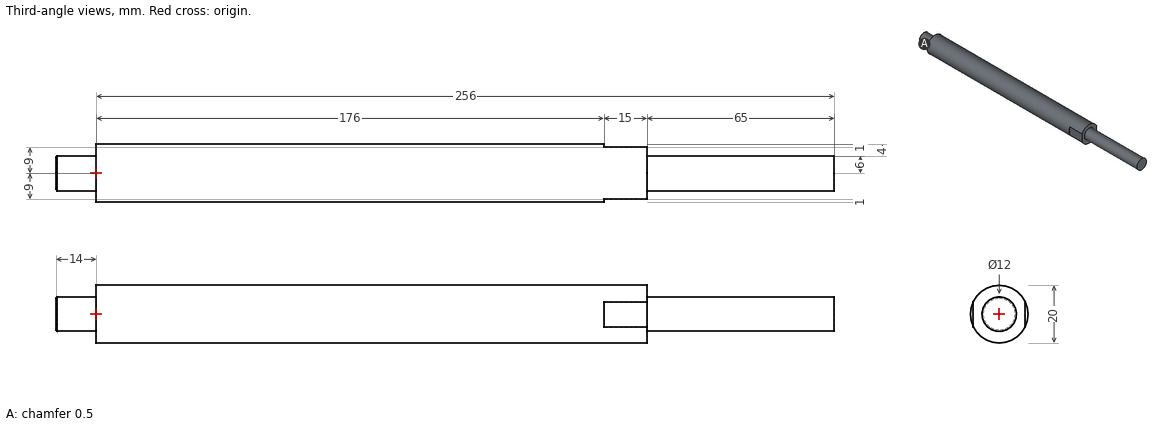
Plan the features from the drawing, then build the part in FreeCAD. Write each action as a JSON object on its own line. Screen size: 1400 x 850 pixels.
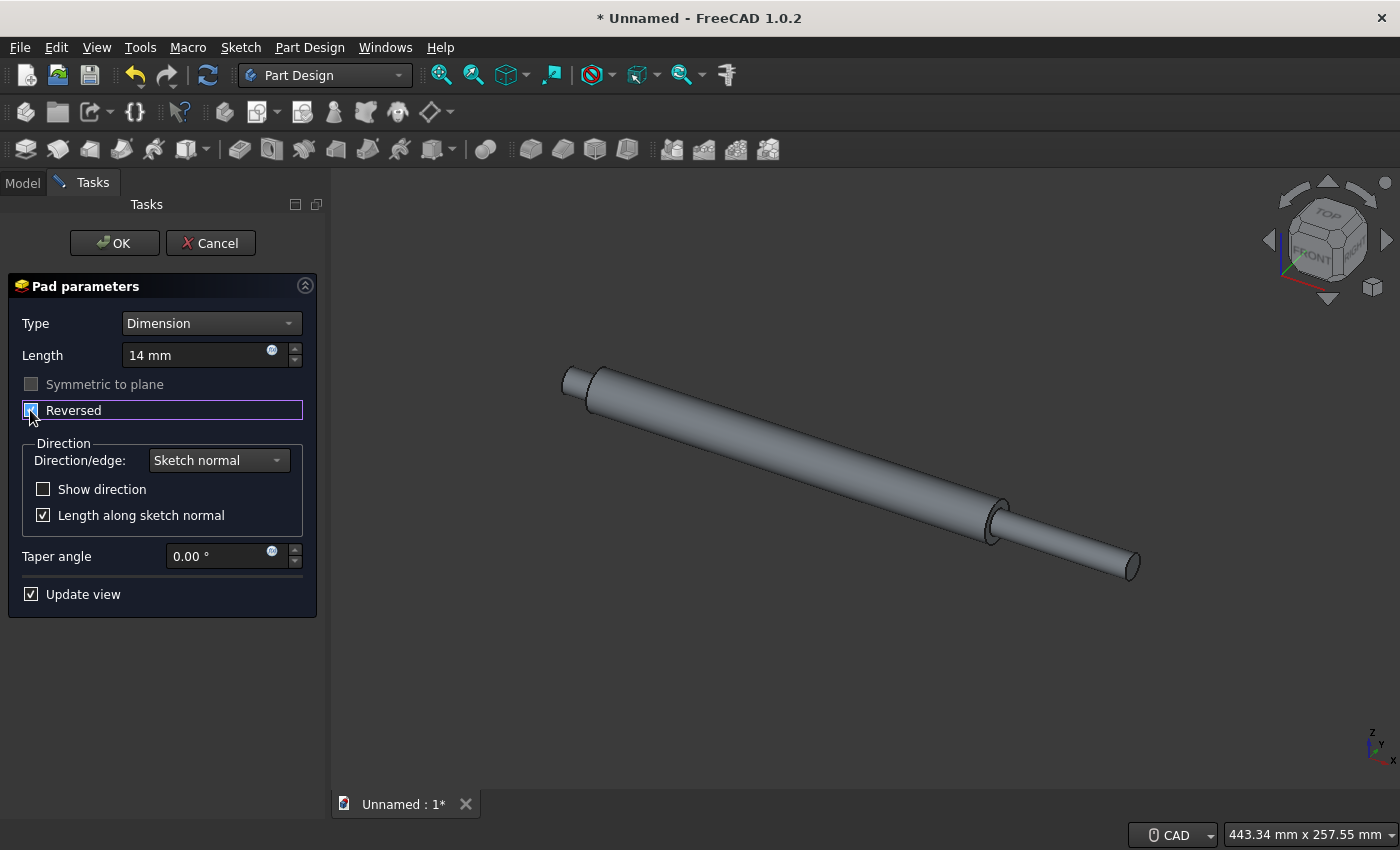
{"action": "left_click", "coordinate": [115, 243]}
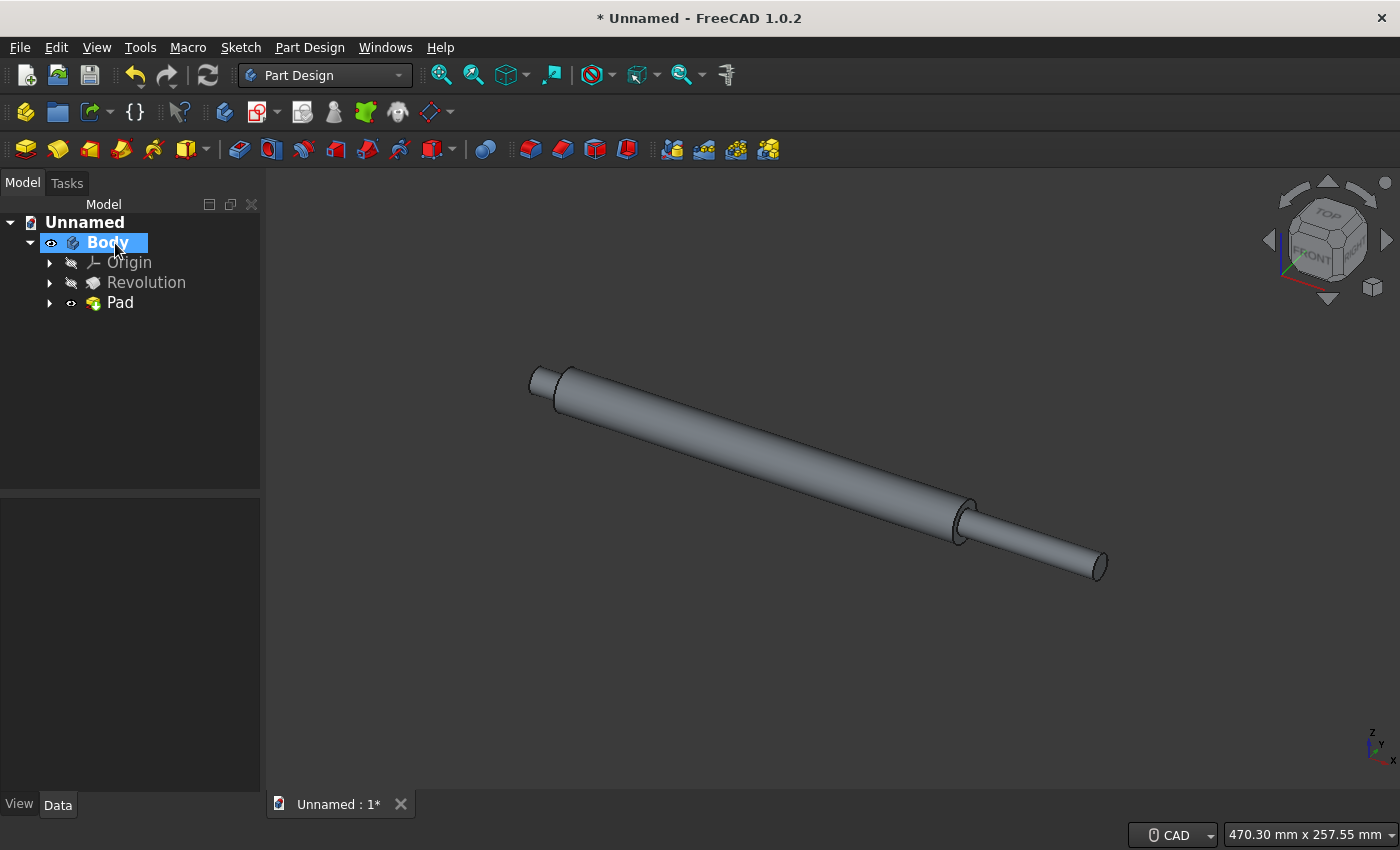
{"action": "left_click", "coordinate": [529, 386]}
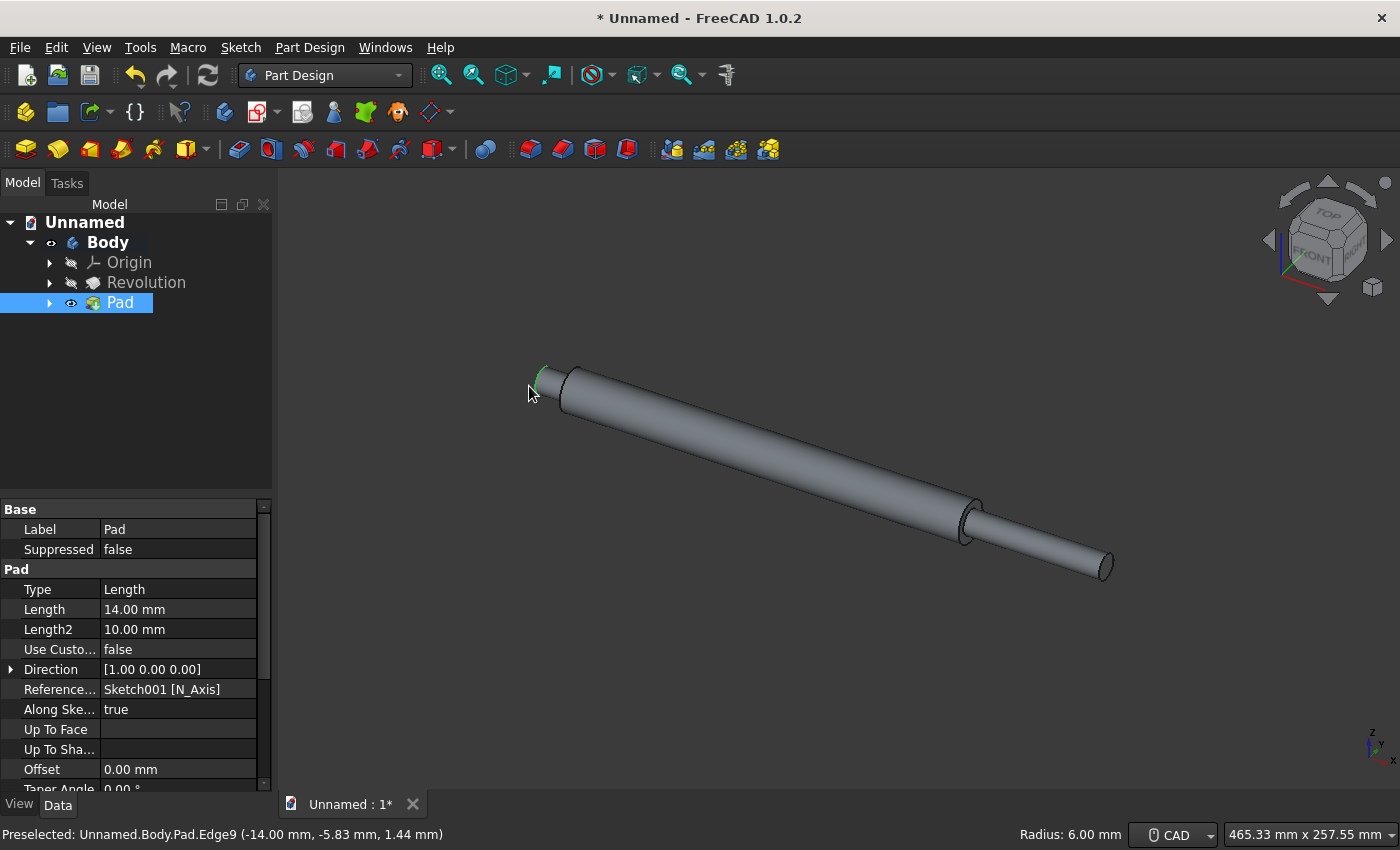
{"action": "left_click", "coordinate": [564, 150]}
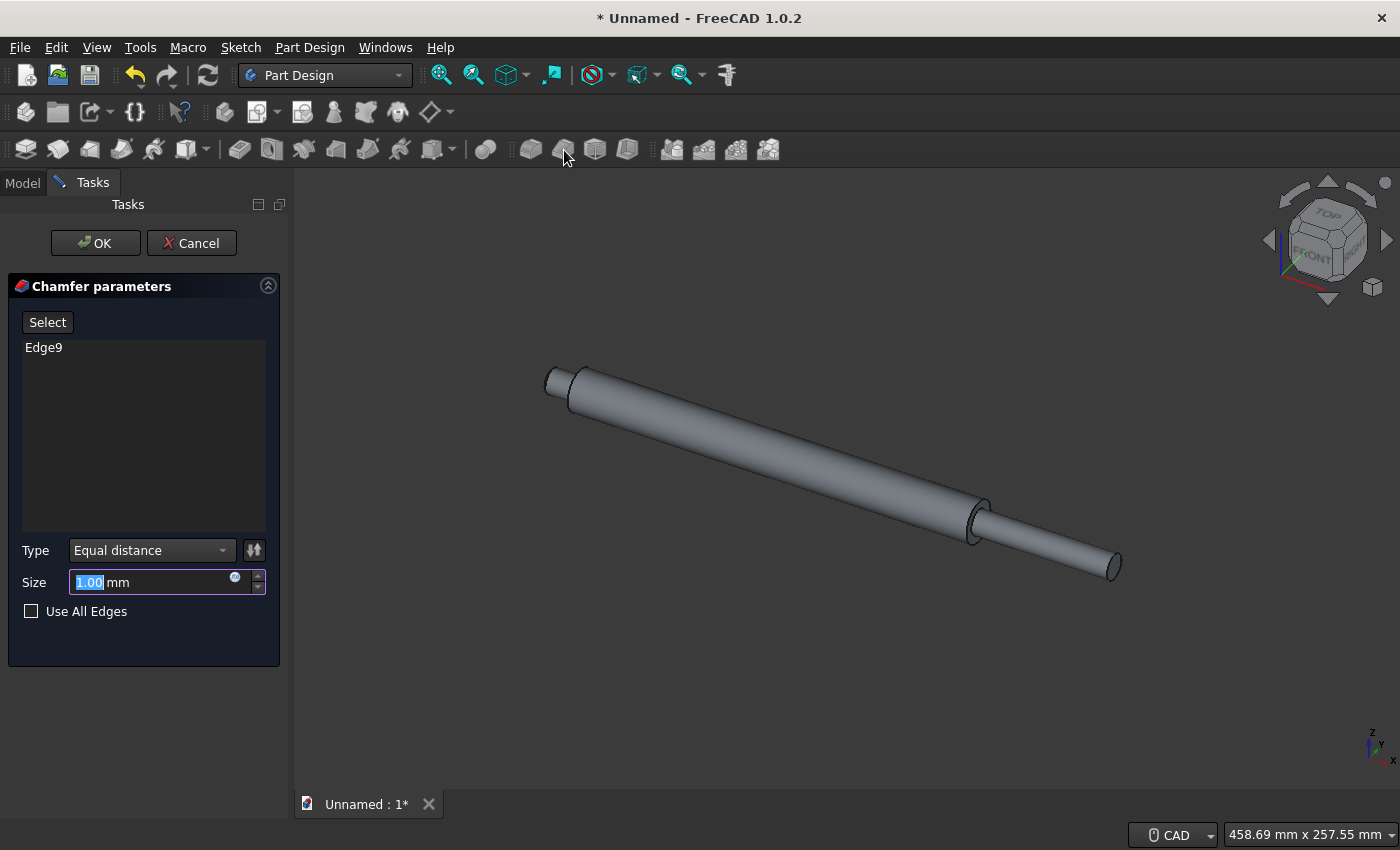
{"action": "type", "text": "0.5"}
{"action": "key", "text": "Tab"}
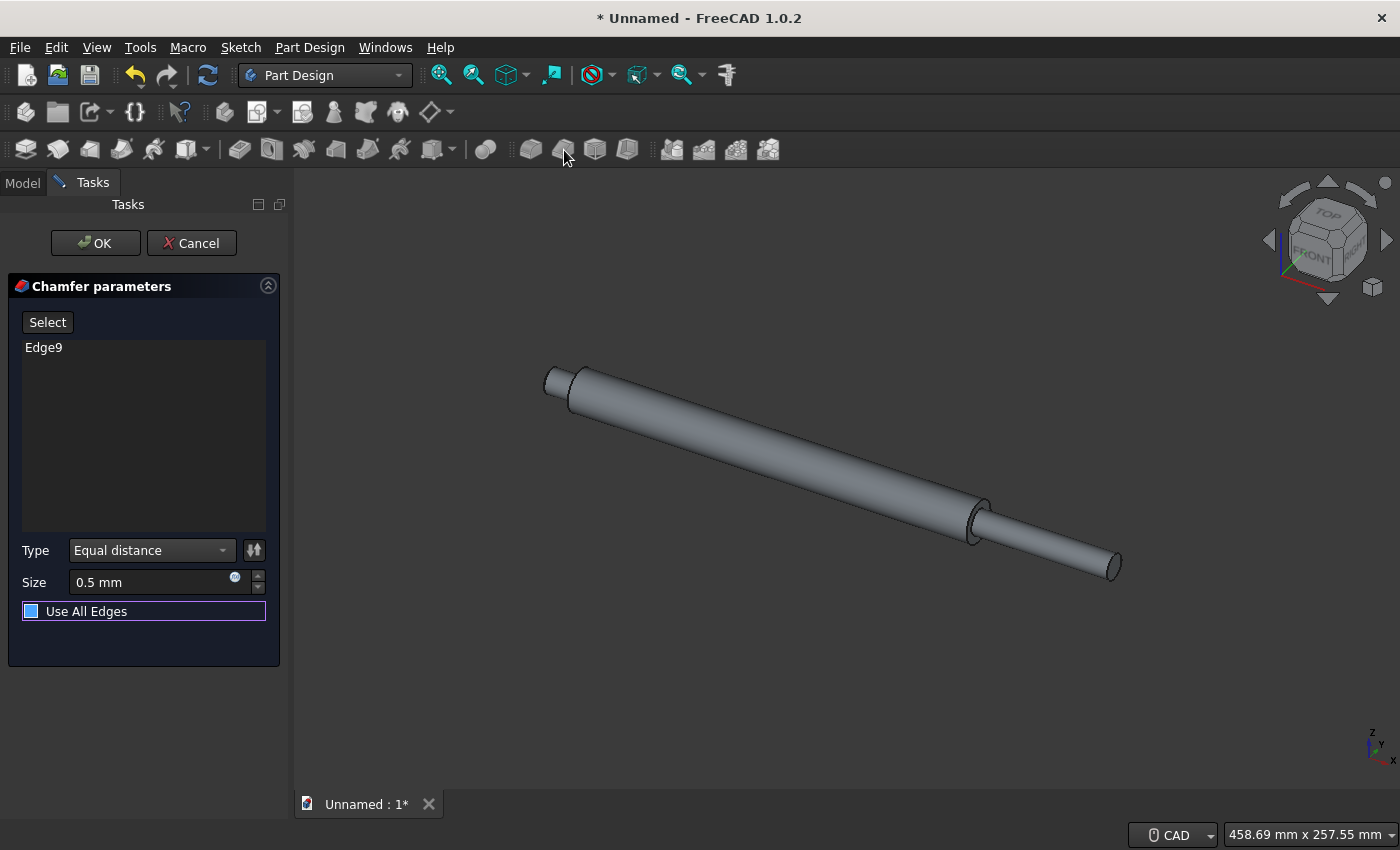
{"action": "left_click", "coordinate": [96, 243]}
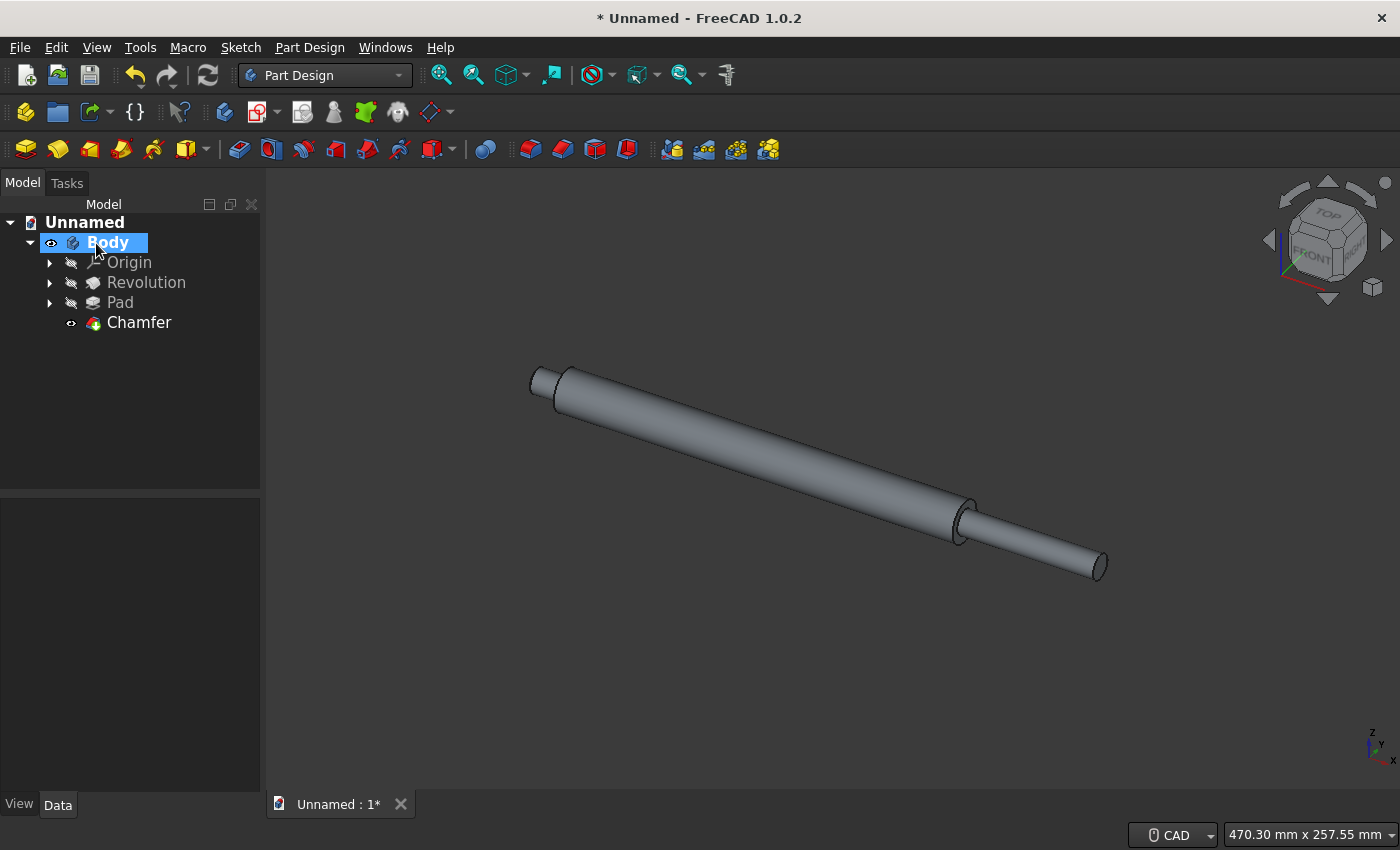
{"action": "left_click", "coordinate": [258, 112]}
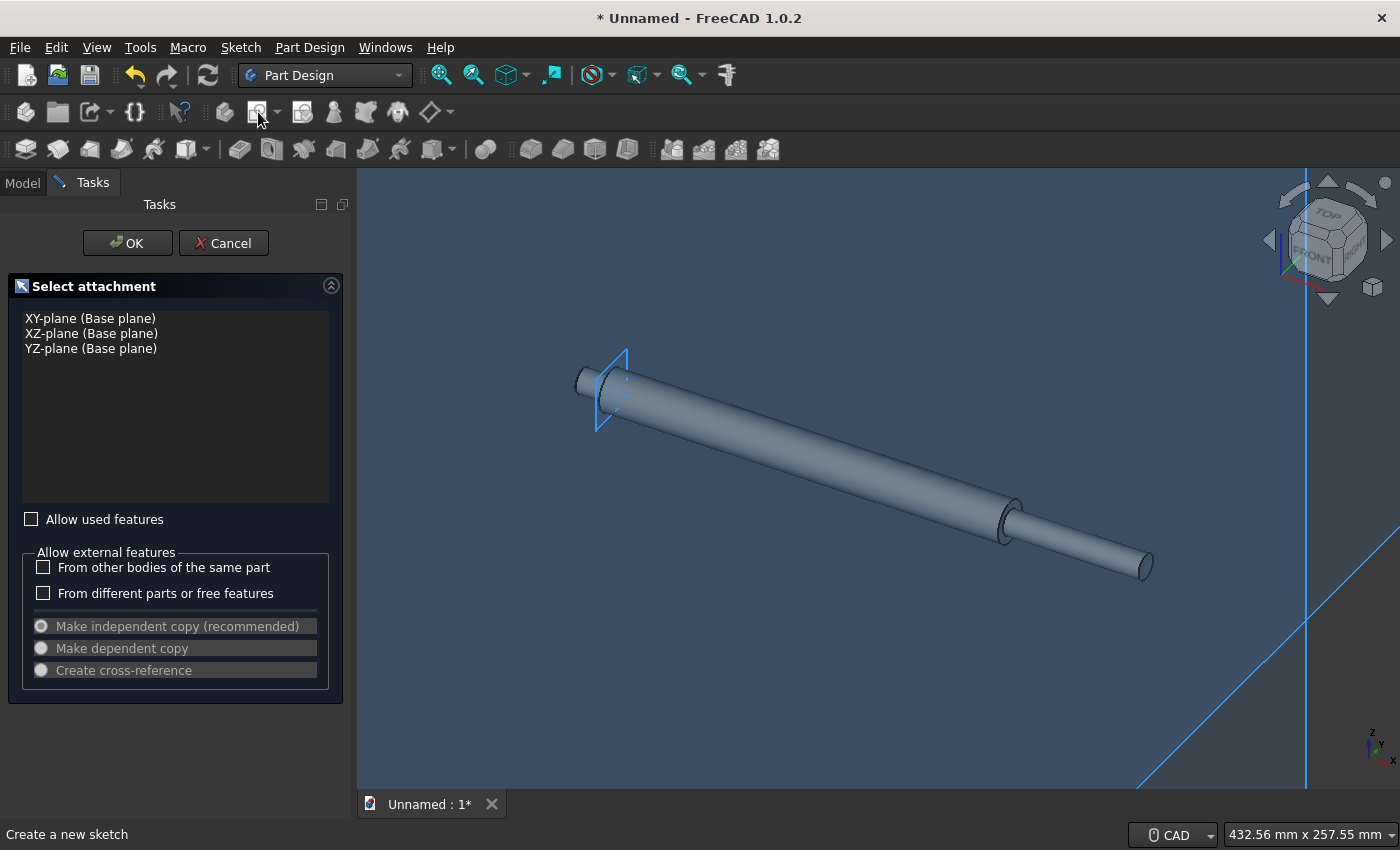
{"action": "left_click", "coordinate": [82, 318]}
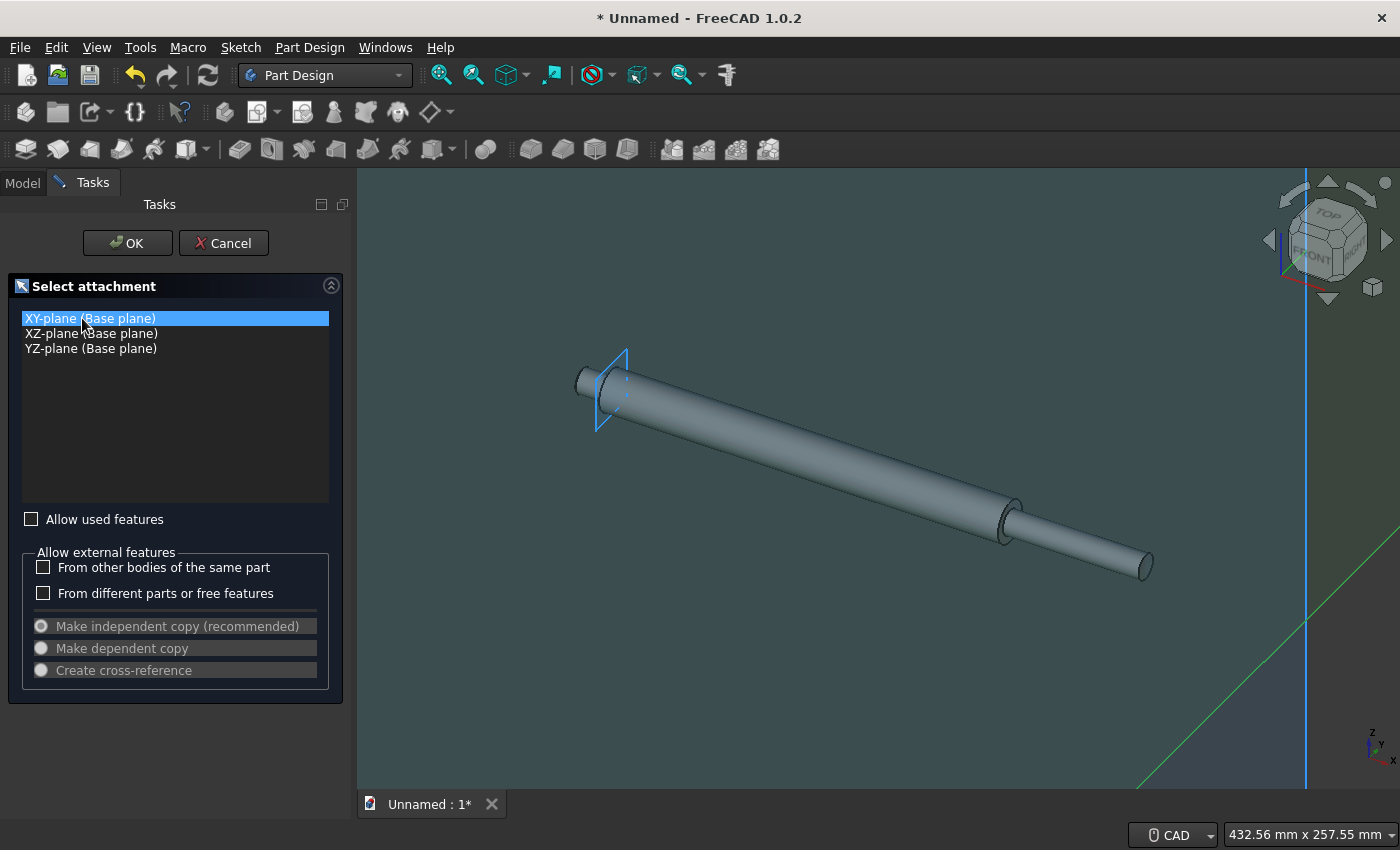
{"action": "left_click", "coordinate": [128, 243]}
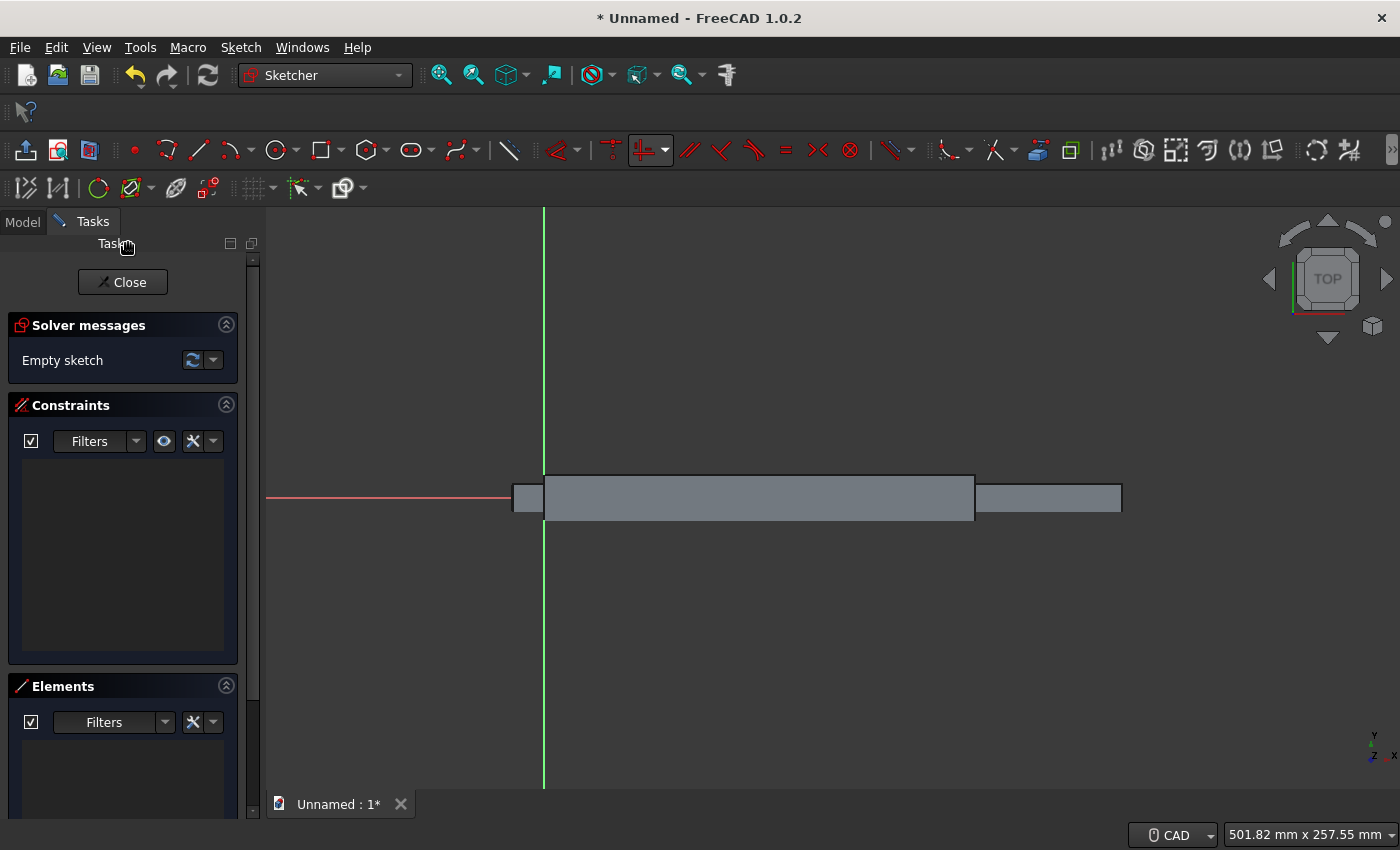
{"action": "key", "text": "q s"}